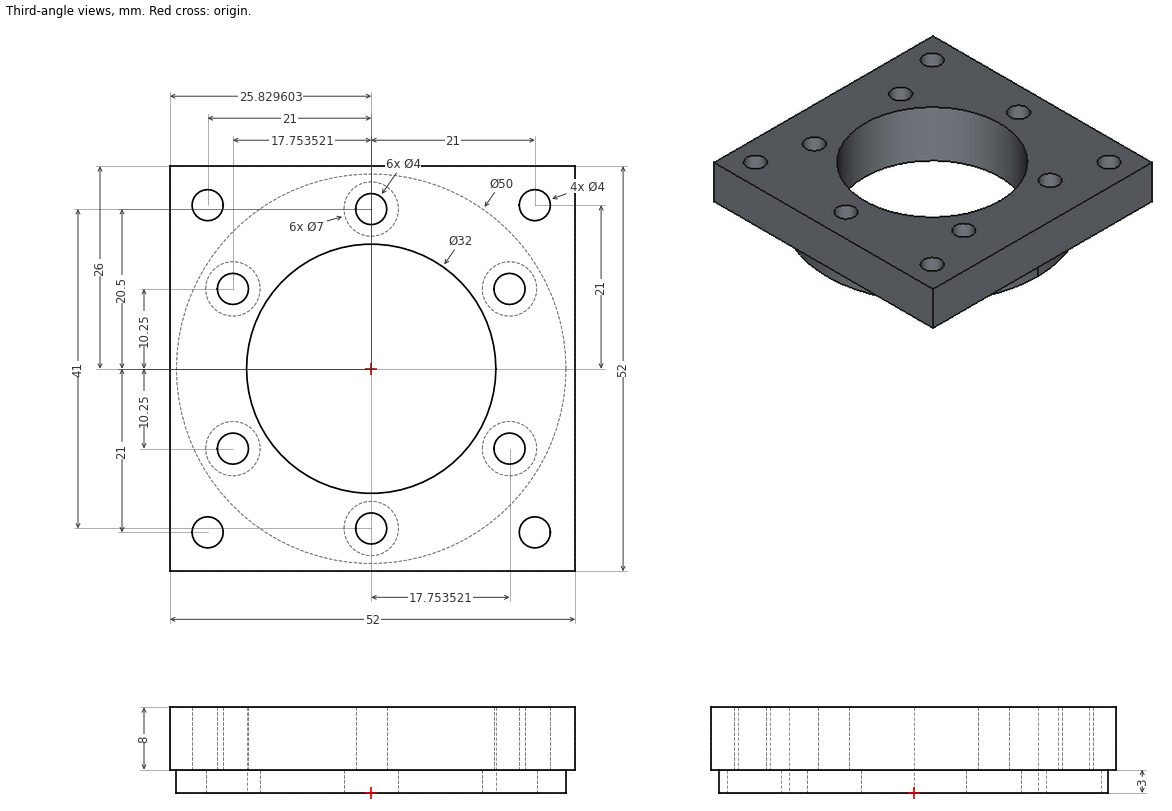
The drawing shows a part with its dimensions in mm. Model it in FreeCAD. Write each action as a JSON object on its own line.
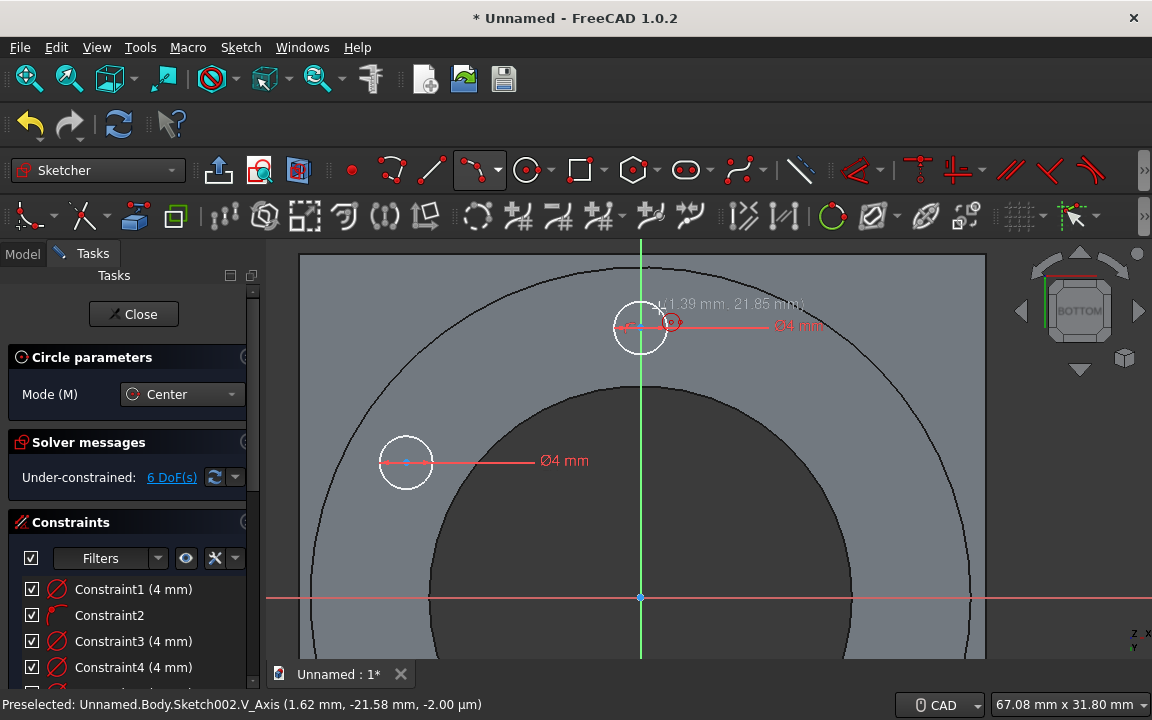
{"action": "left_click", "coordinate": [875, 462]}
{"action": "mouse_move", "coordinate": [894, 443]}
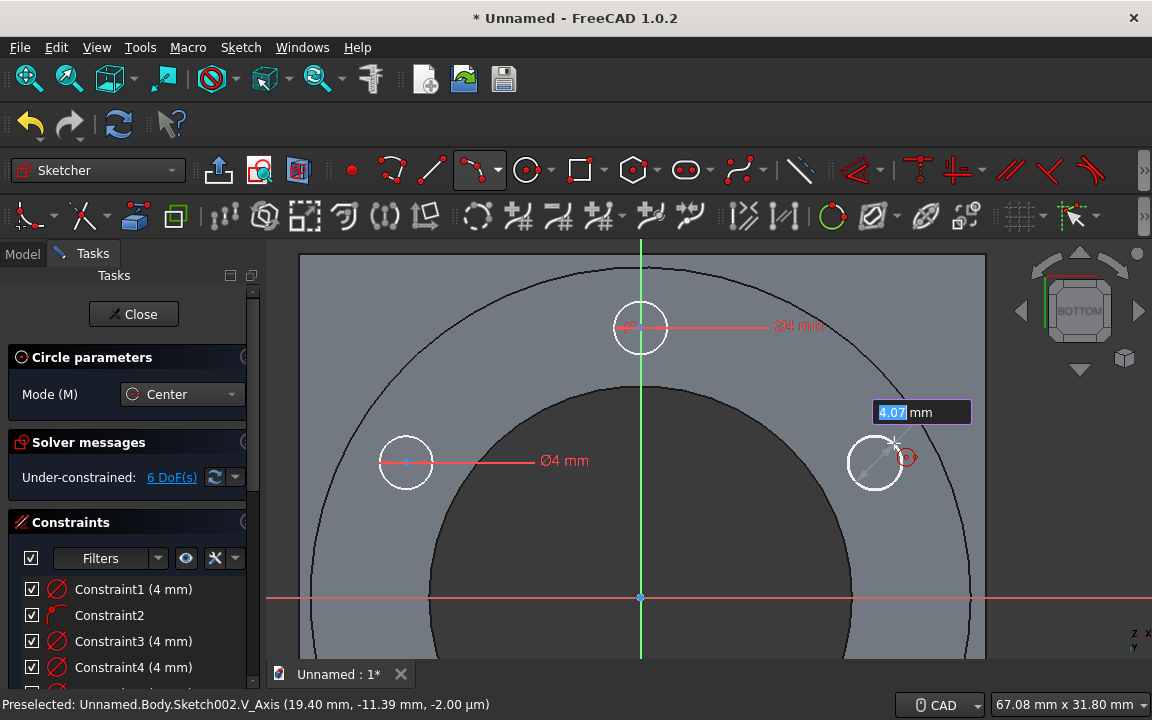
{"action": "type", "text": "4"}
{"action": "key", "text": "Return"}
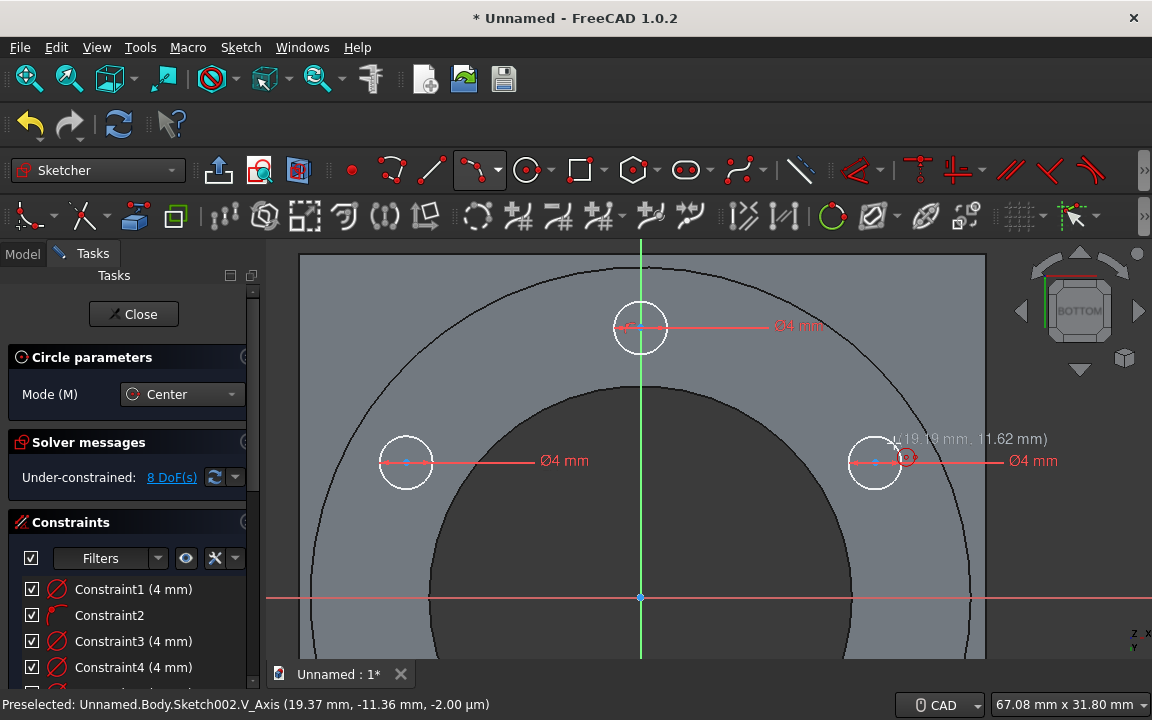
{"action": "scroll", "coordinate": [640, 328], "scroll_direction": "down", "scroll_amount": 4}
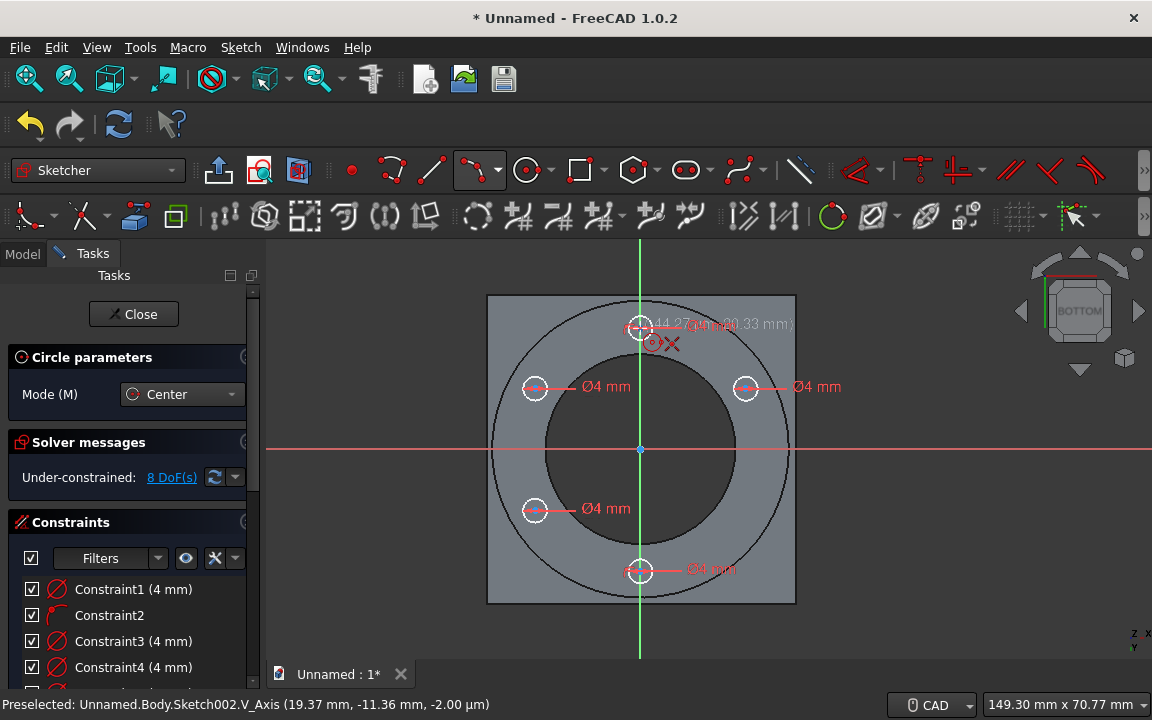
{"action": "scroll", "coordinate": [746, 510], "scroll_direction": "up", "scroll_amount": 4}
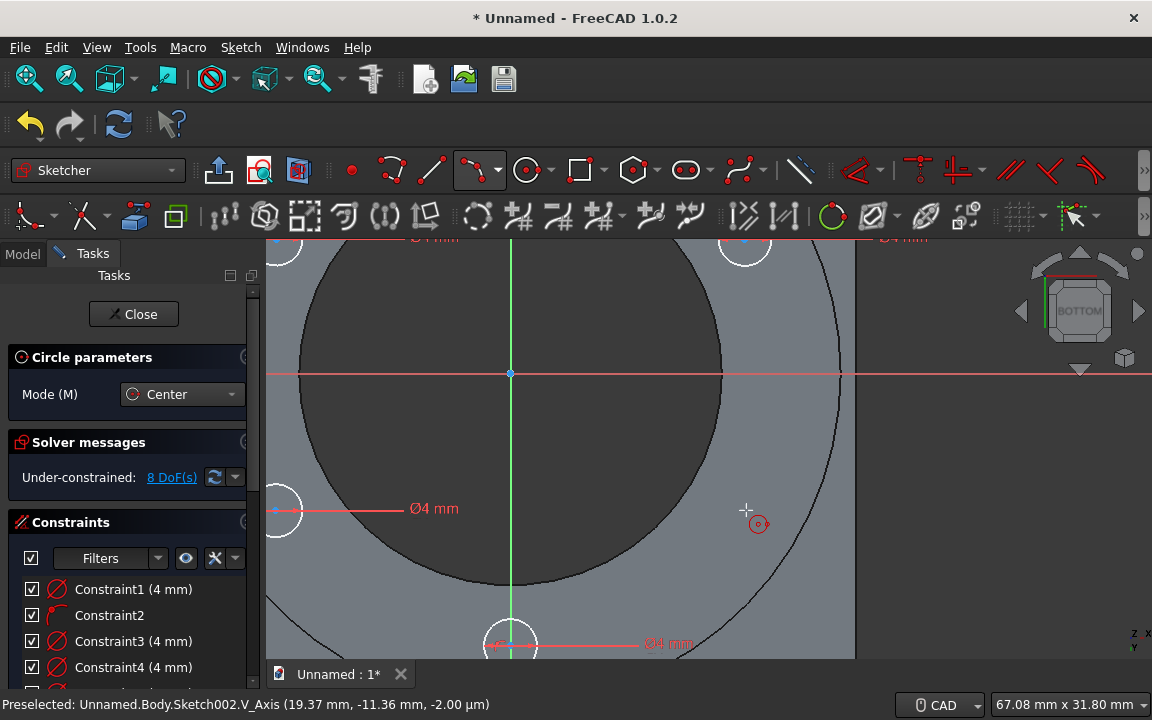
{"action": "left_click", "coordinate": [745, 509]}
{"action": "mouse_move", "coordinate": [764, 491]}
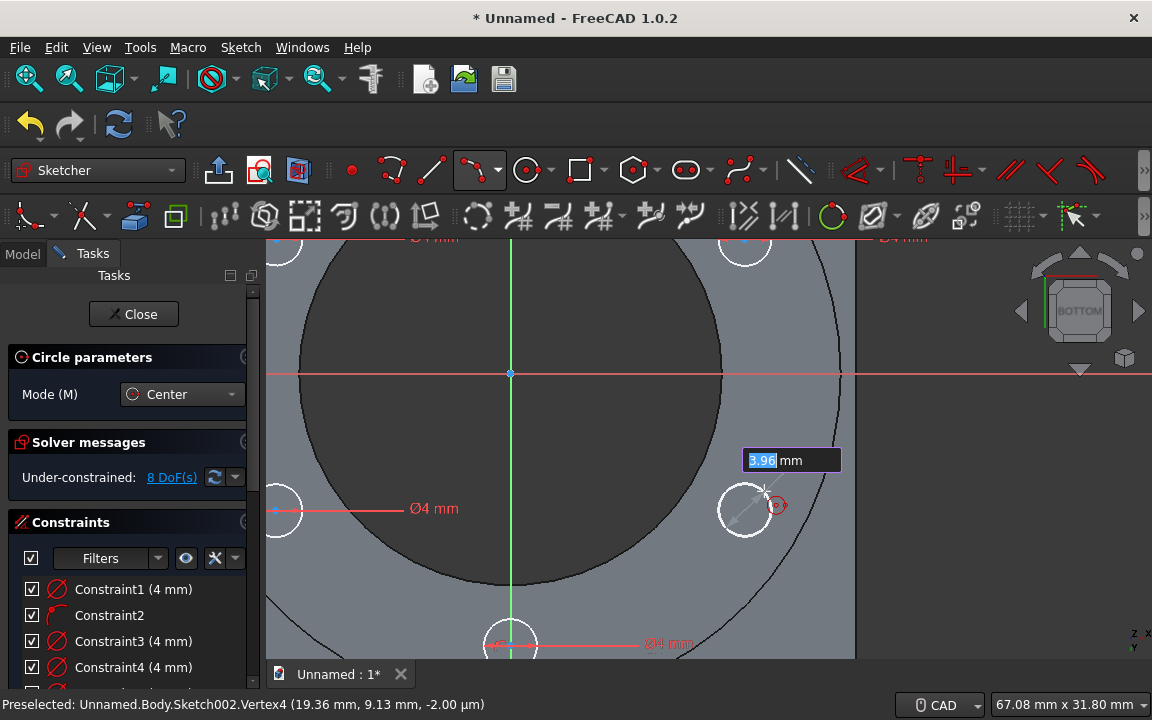
{"action": "type", "text": "4"}
{"action": "key", "text": "Return"}
{"action": "key", "text": "Escape"}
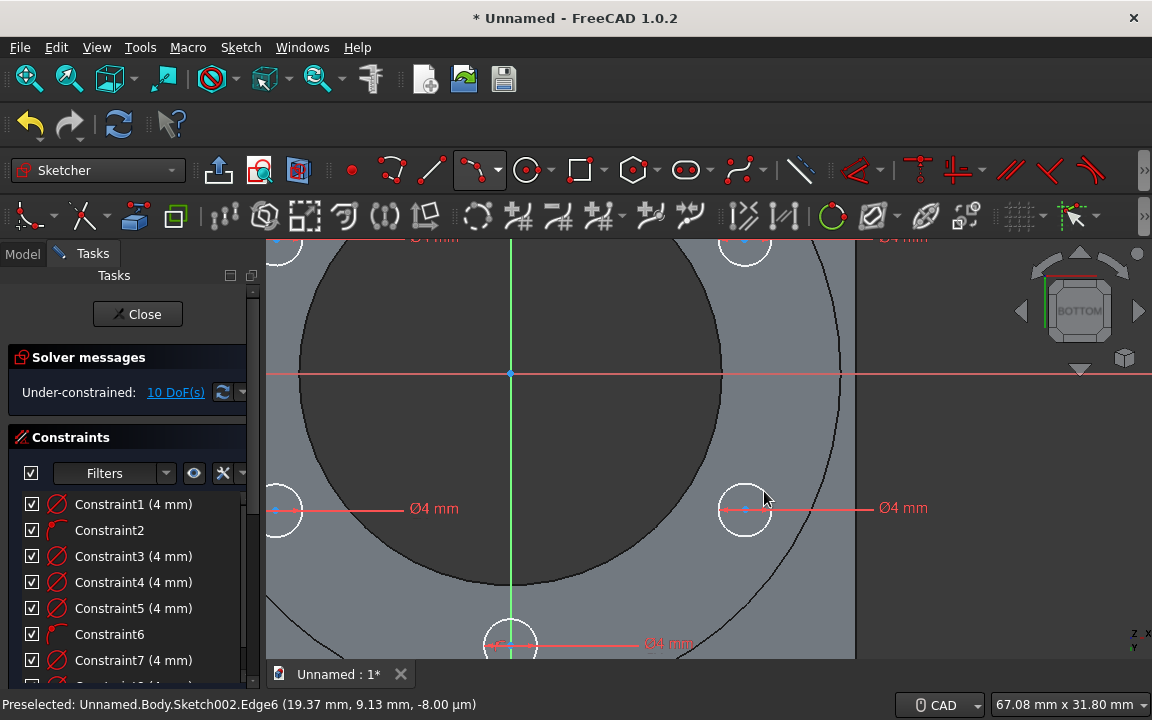
{"action": "scroll", "coordinate": [747, 510], "scroll_direction": "down", "scroll_amount": 4}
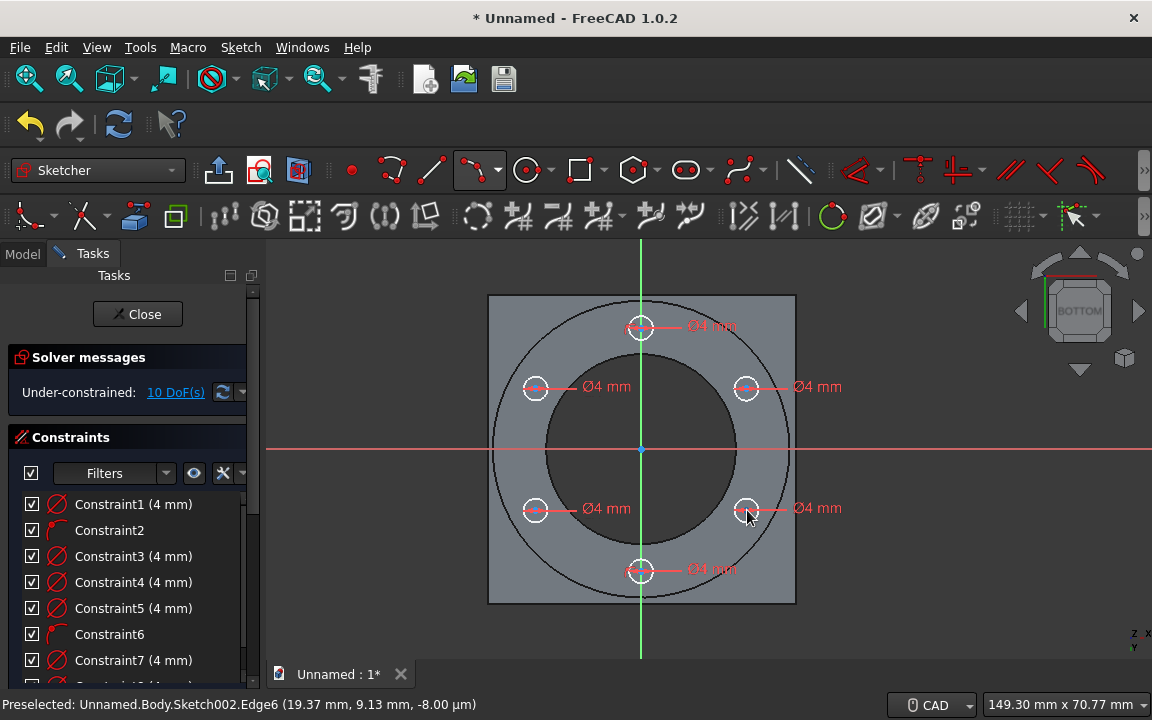
{"action": "left_click", "coordinate": [536, 511]}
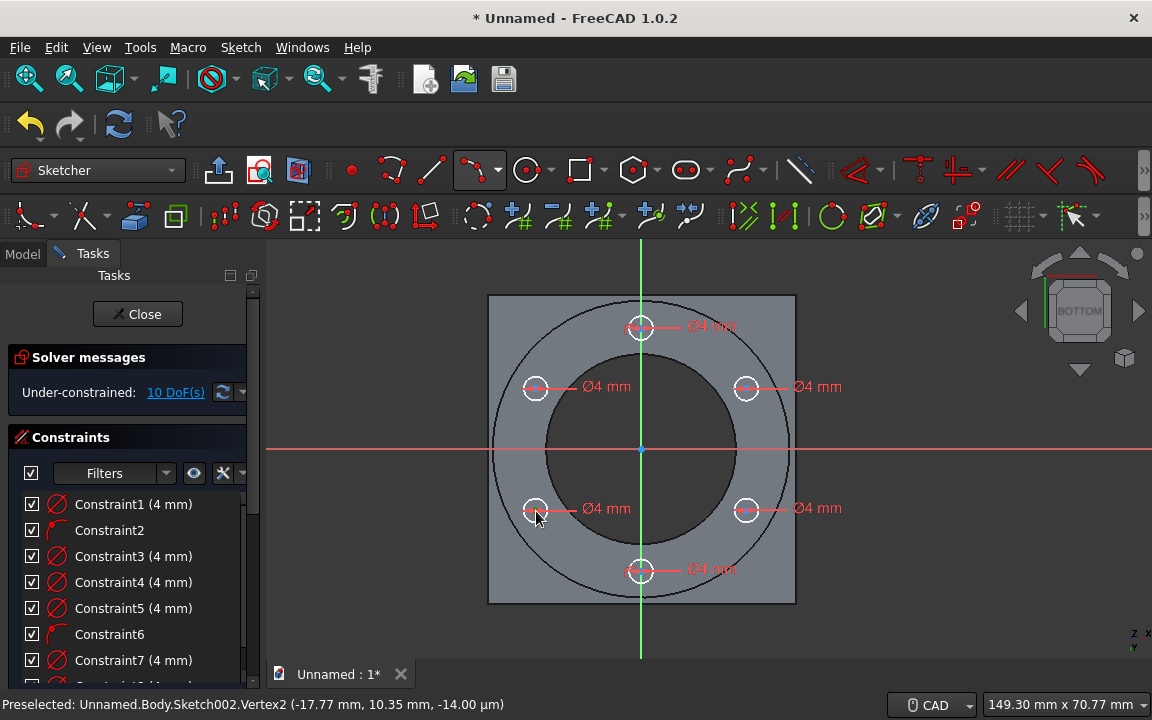
{"action": "left_click", "coordinate": [536, 389]}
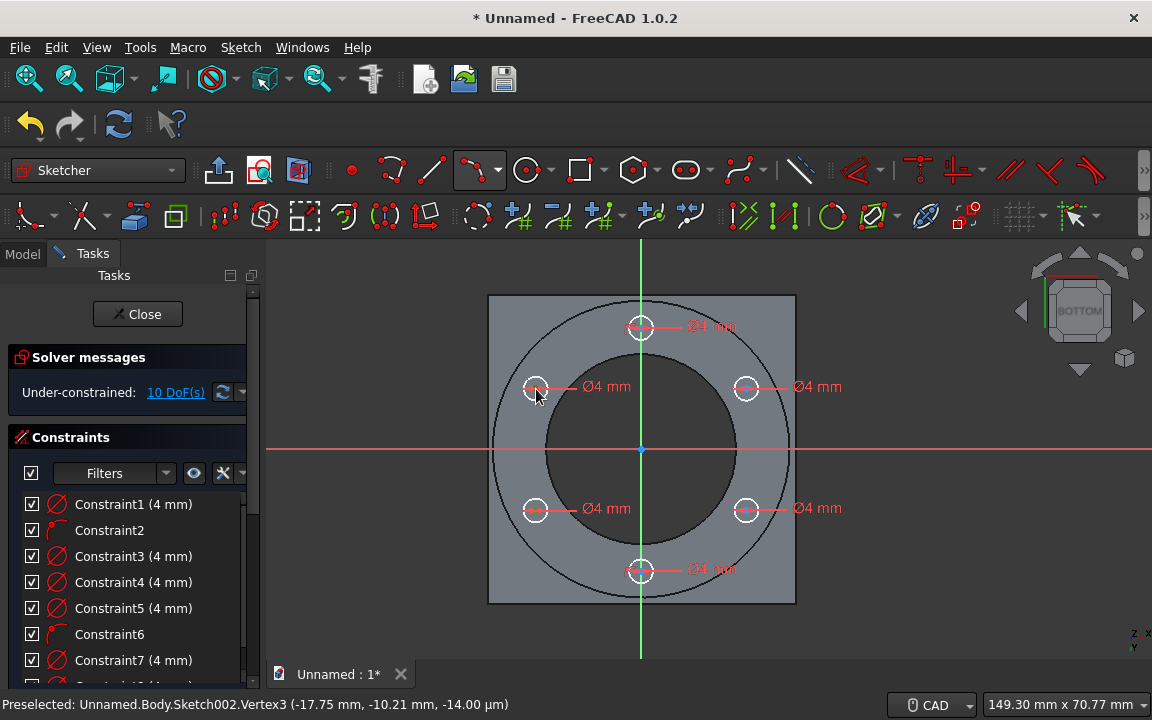
{"action": "key", "text": "v"}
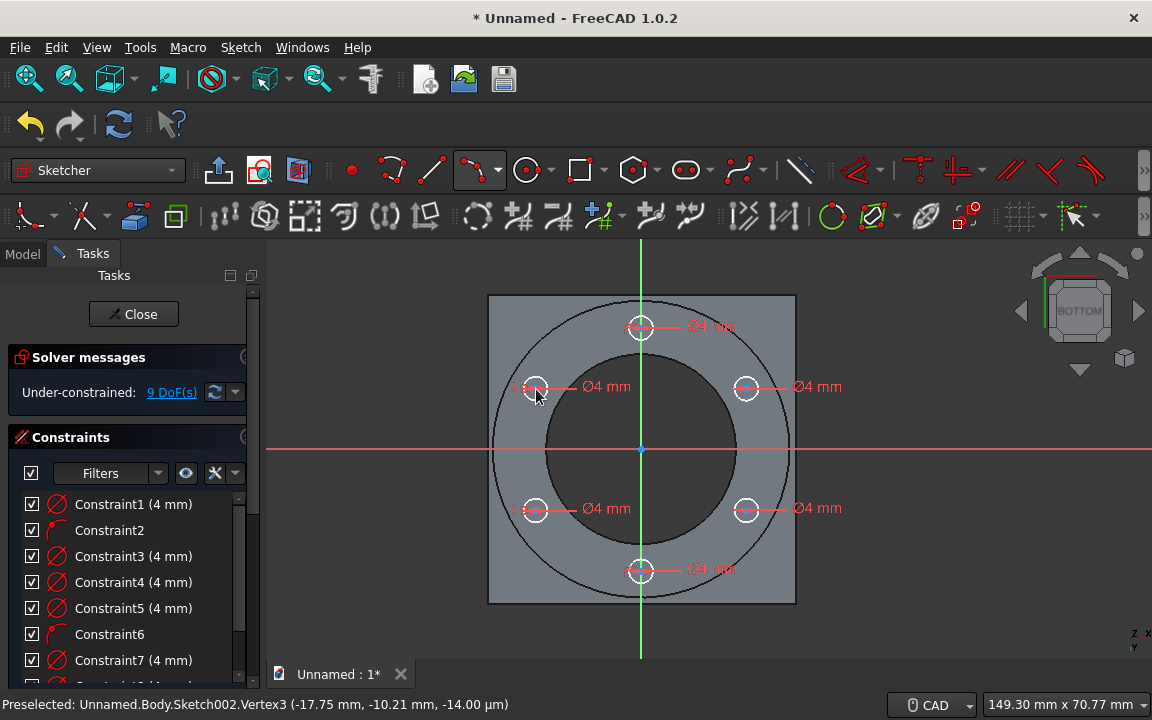
{"action": "left_click", "coordinate": [536, 389]}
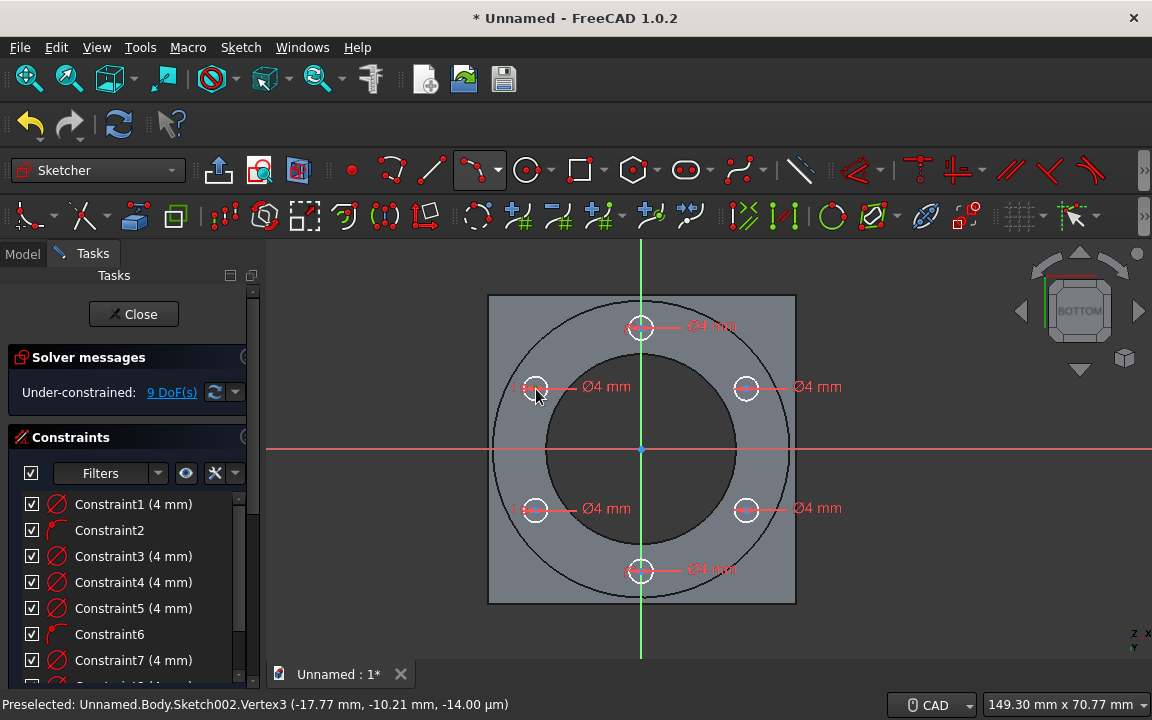
{"action": "left_click", "coordinate": [746, 389]}